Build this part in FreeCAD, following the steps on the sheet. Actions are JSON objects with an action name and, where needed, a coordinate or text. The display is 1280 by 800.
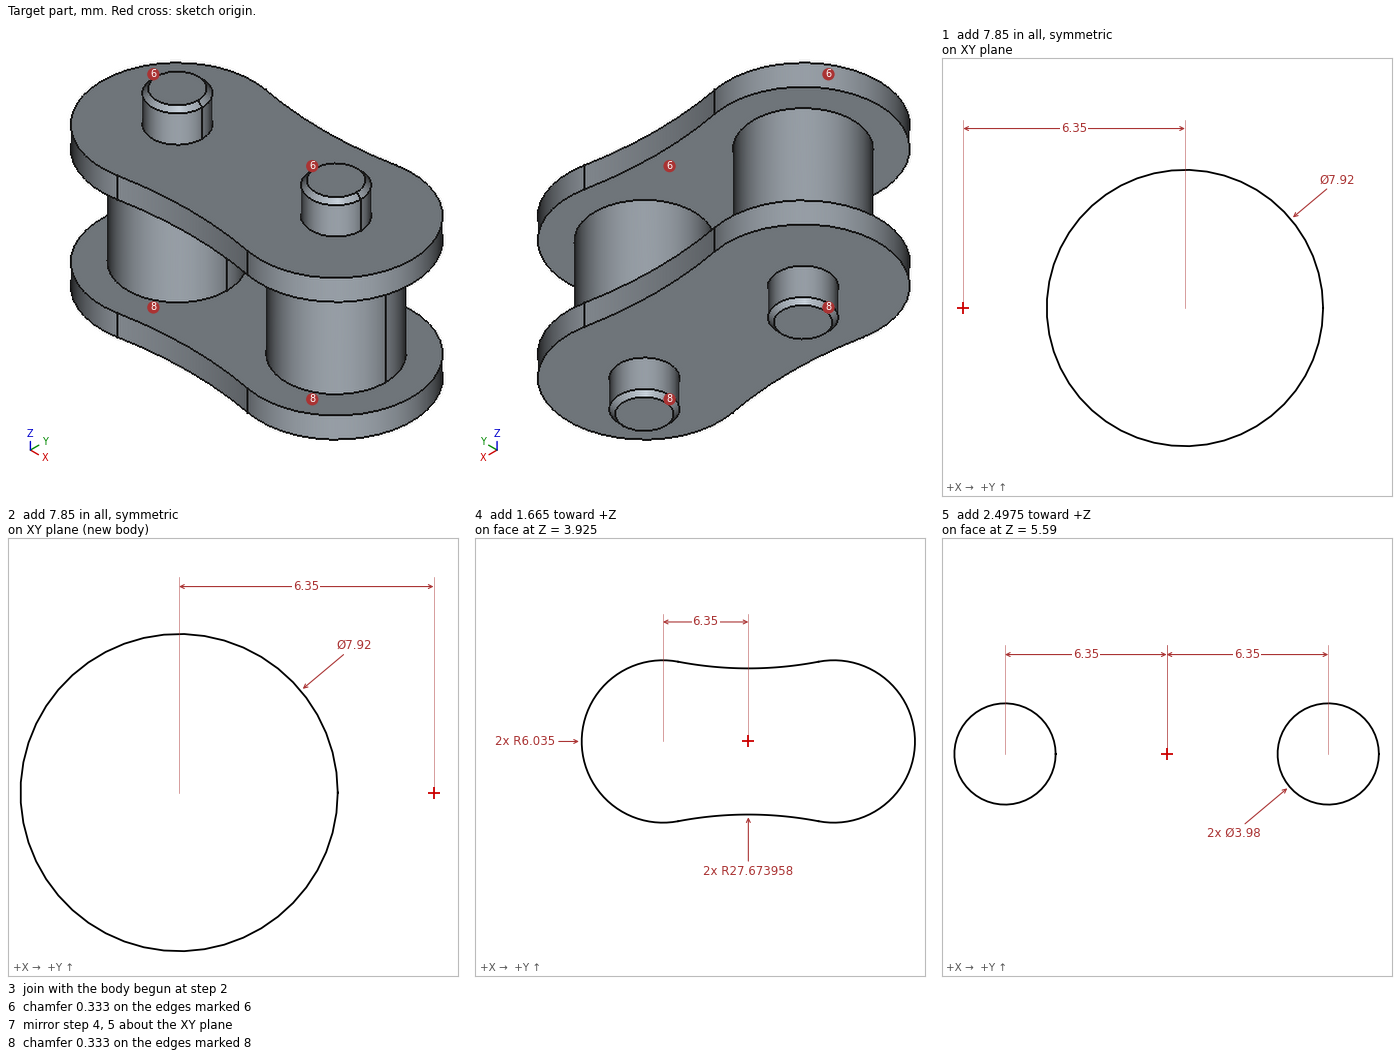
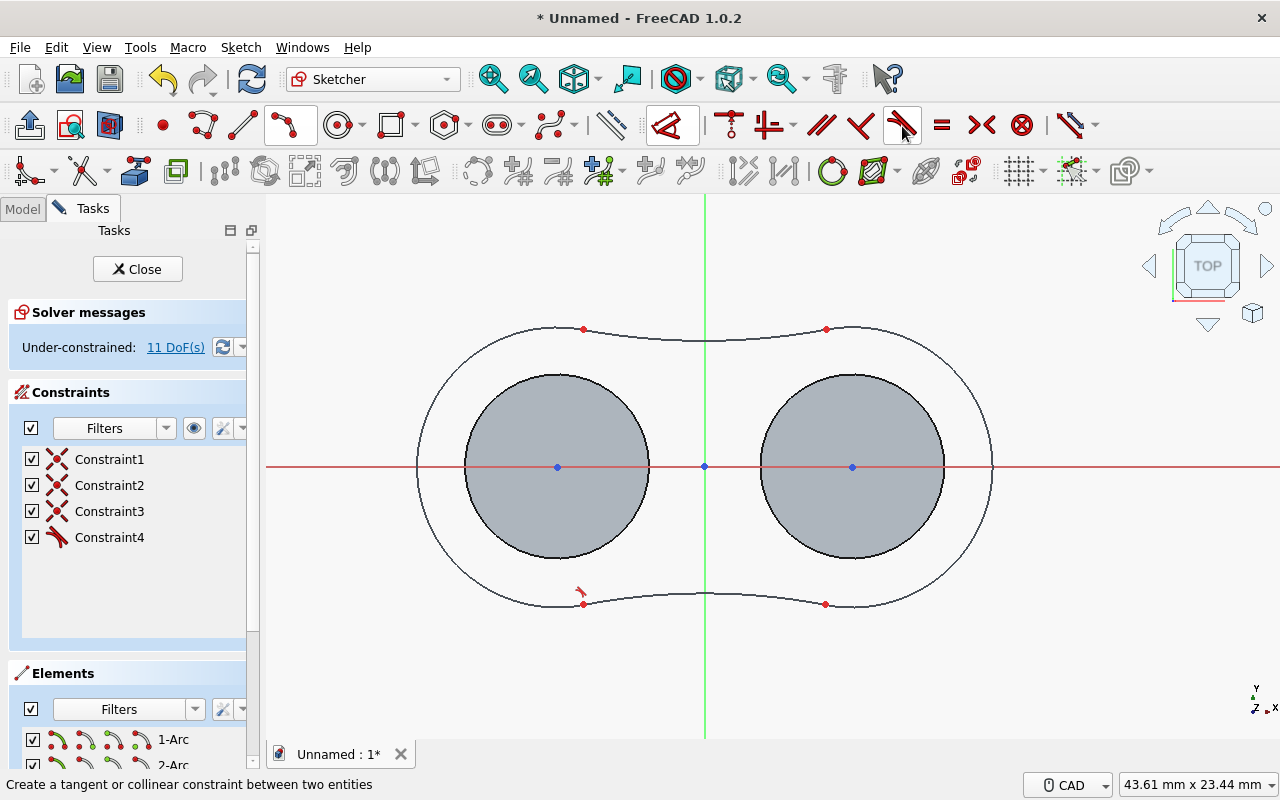
{"action": "left_click", "coordinate": [450, 377]}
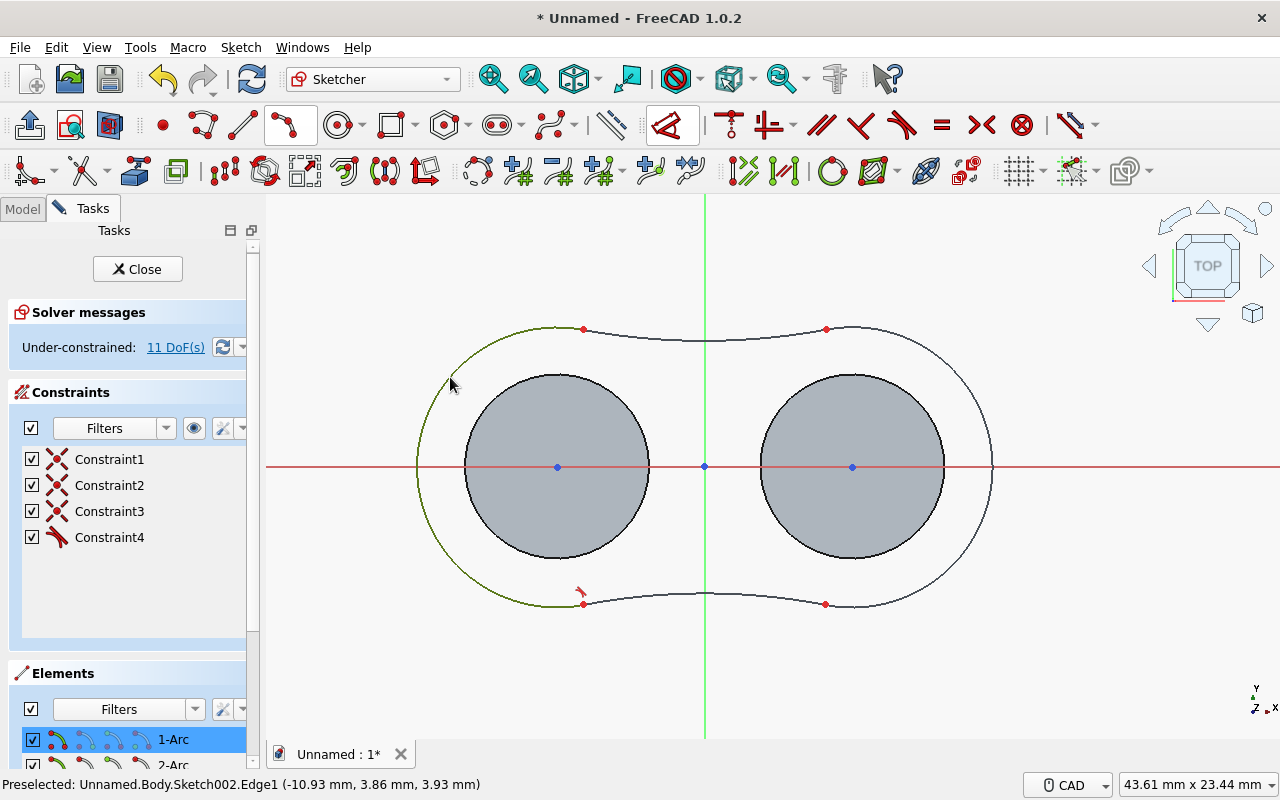
{"action": "left_click", "coordinate": [656, 339]}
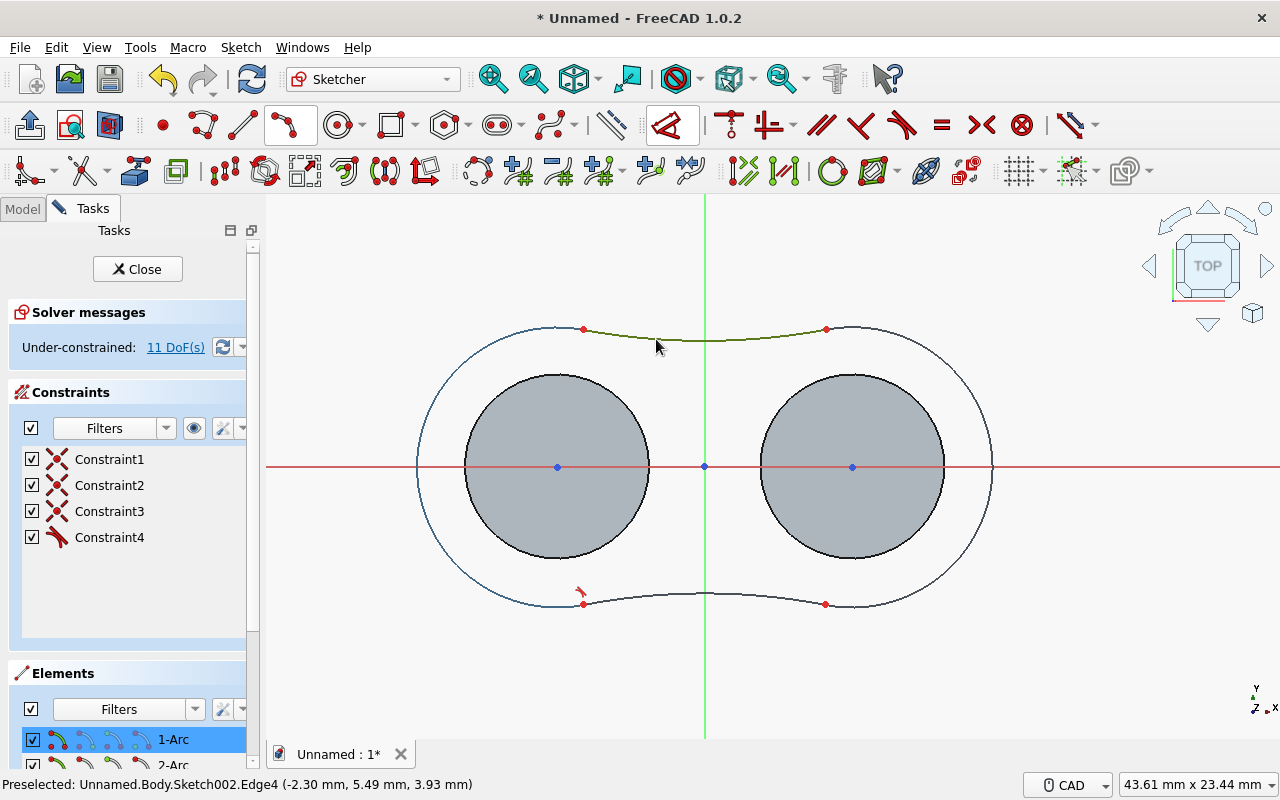
{"action": "key", "text": "t"}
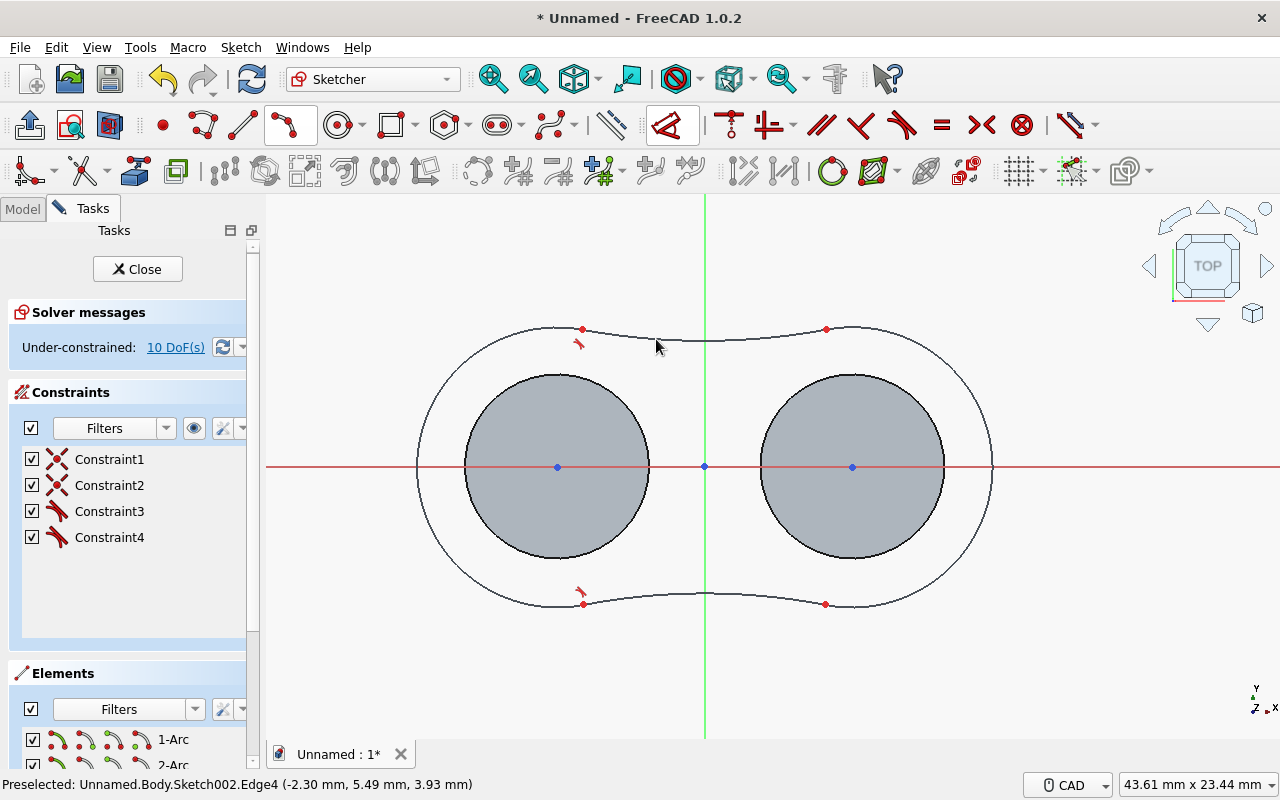
{"action": "left_click", "coordinate": [753, 595]}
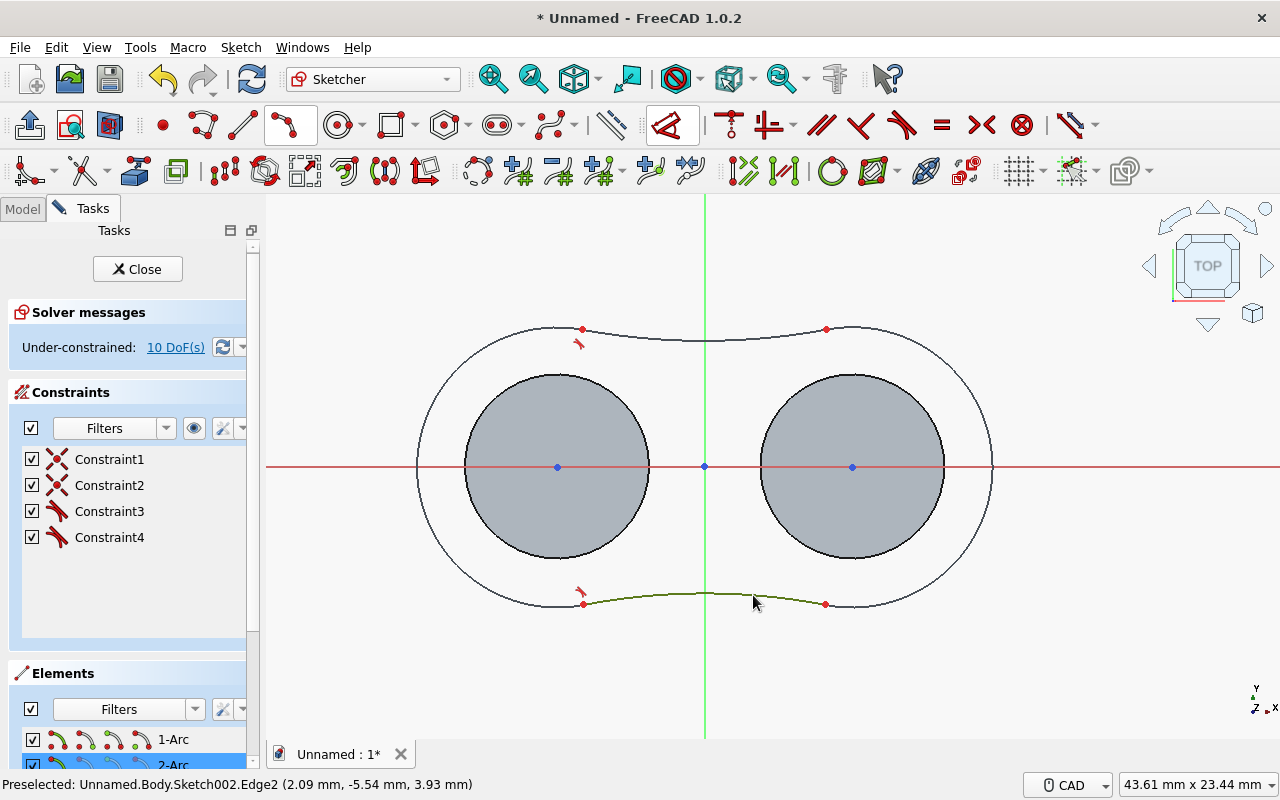
{"action": "left_click", "coordinate": [959, 558]}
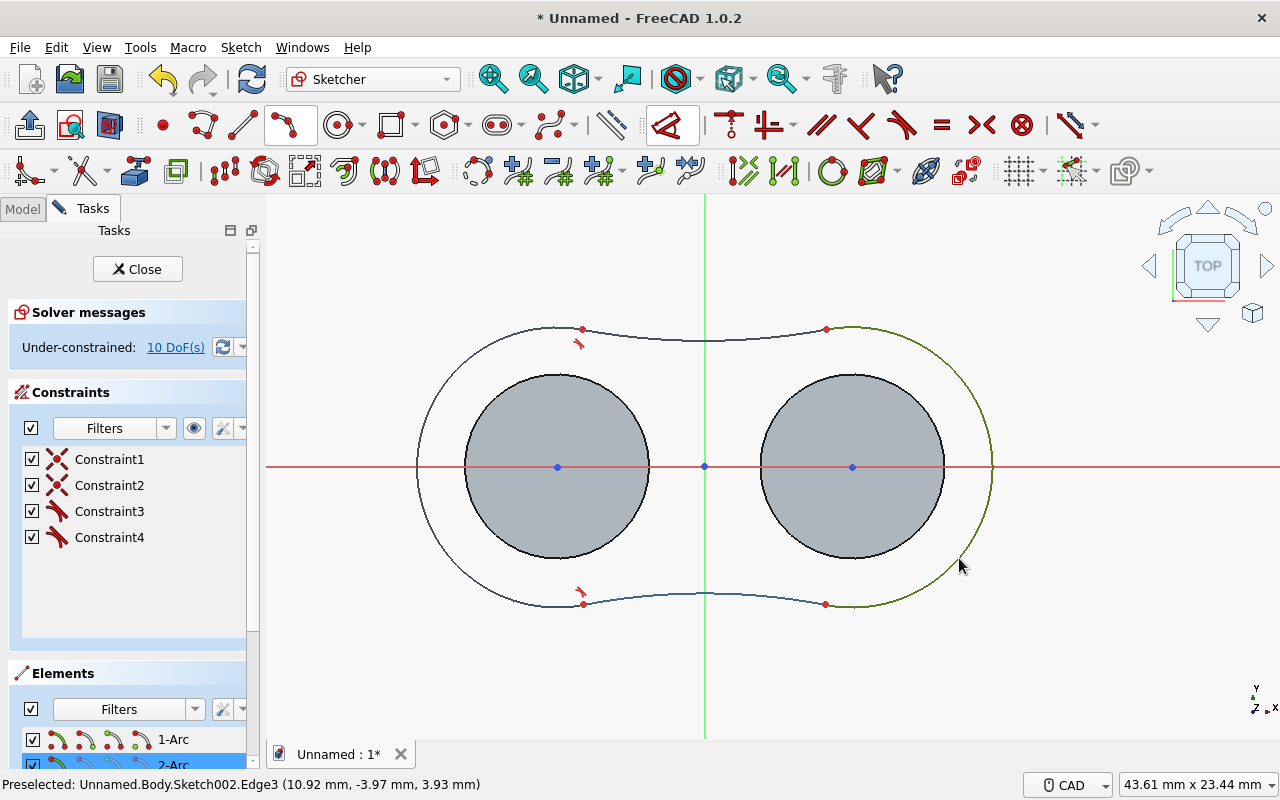
{"action": "key", "text": "t"}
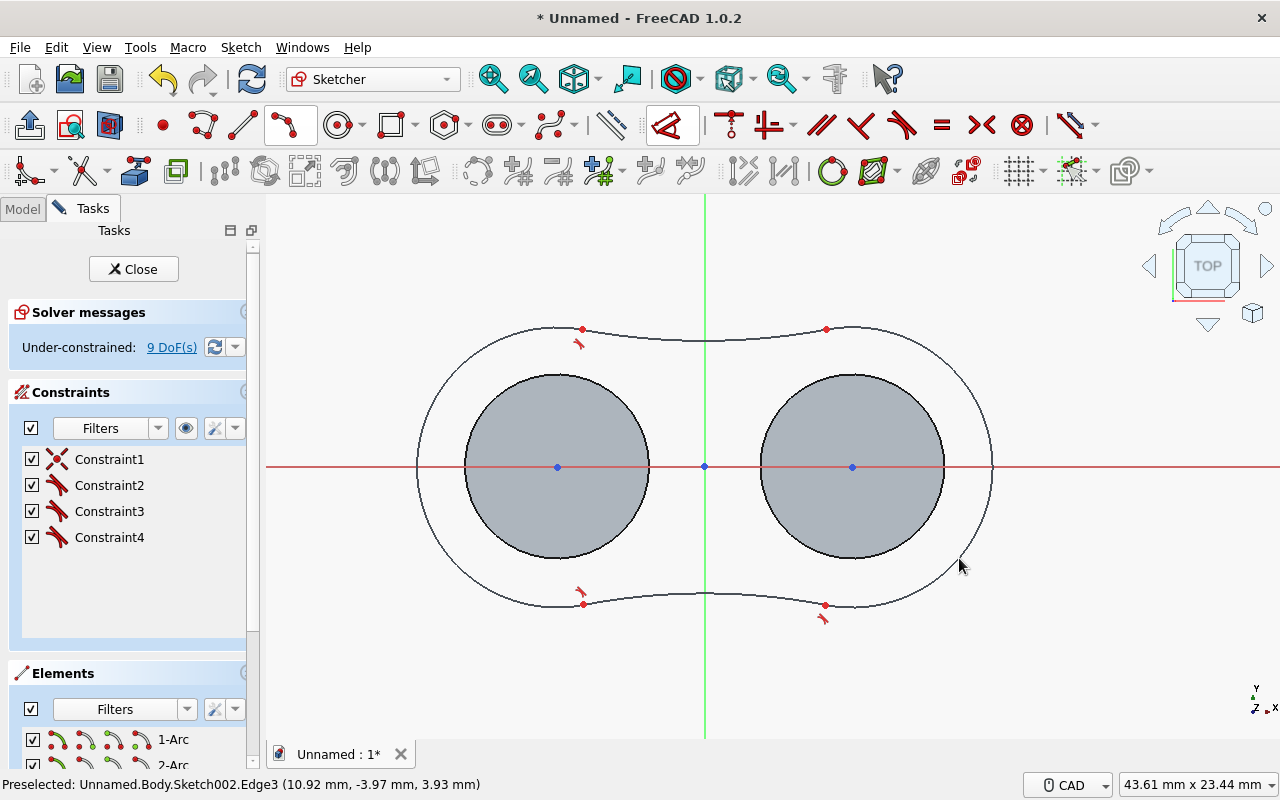
{"action": "left_click", "coordinate": [959, 558]}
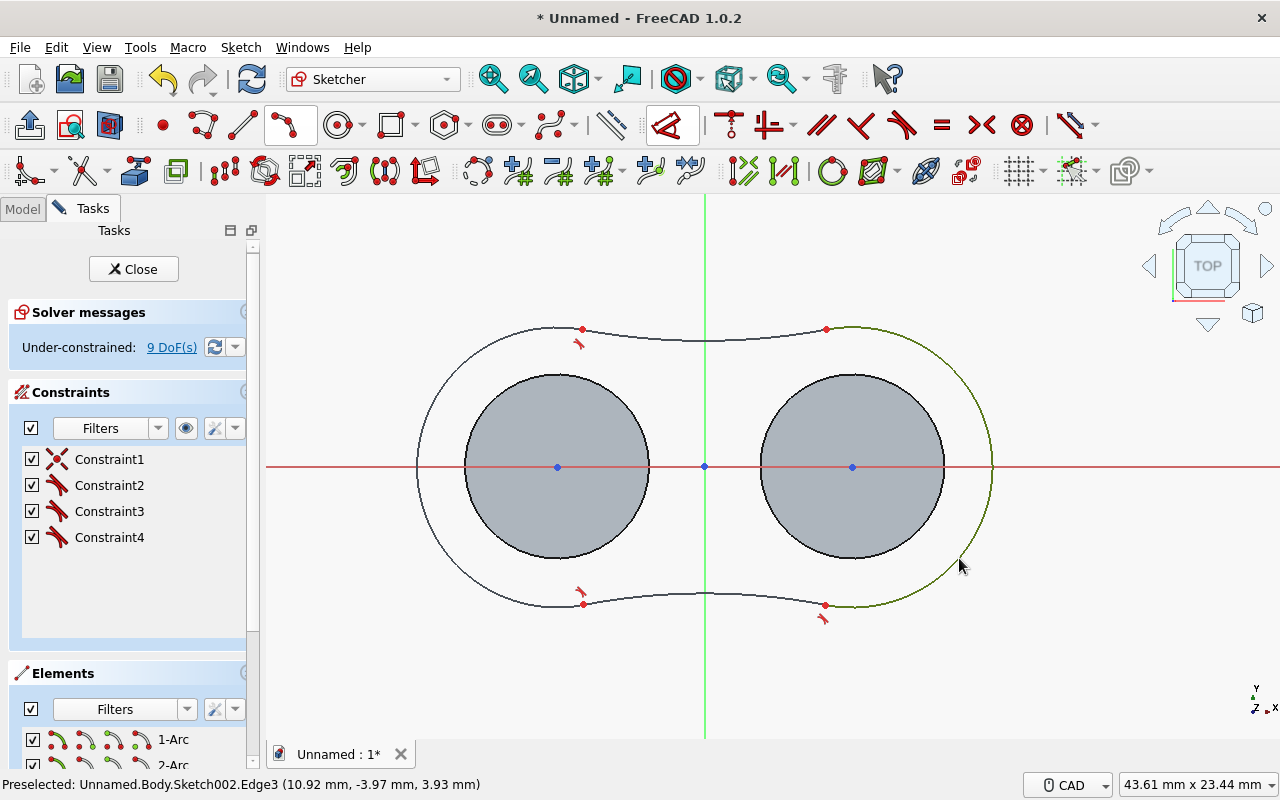
{"action": "left_click", "coordinate": [655, 339]}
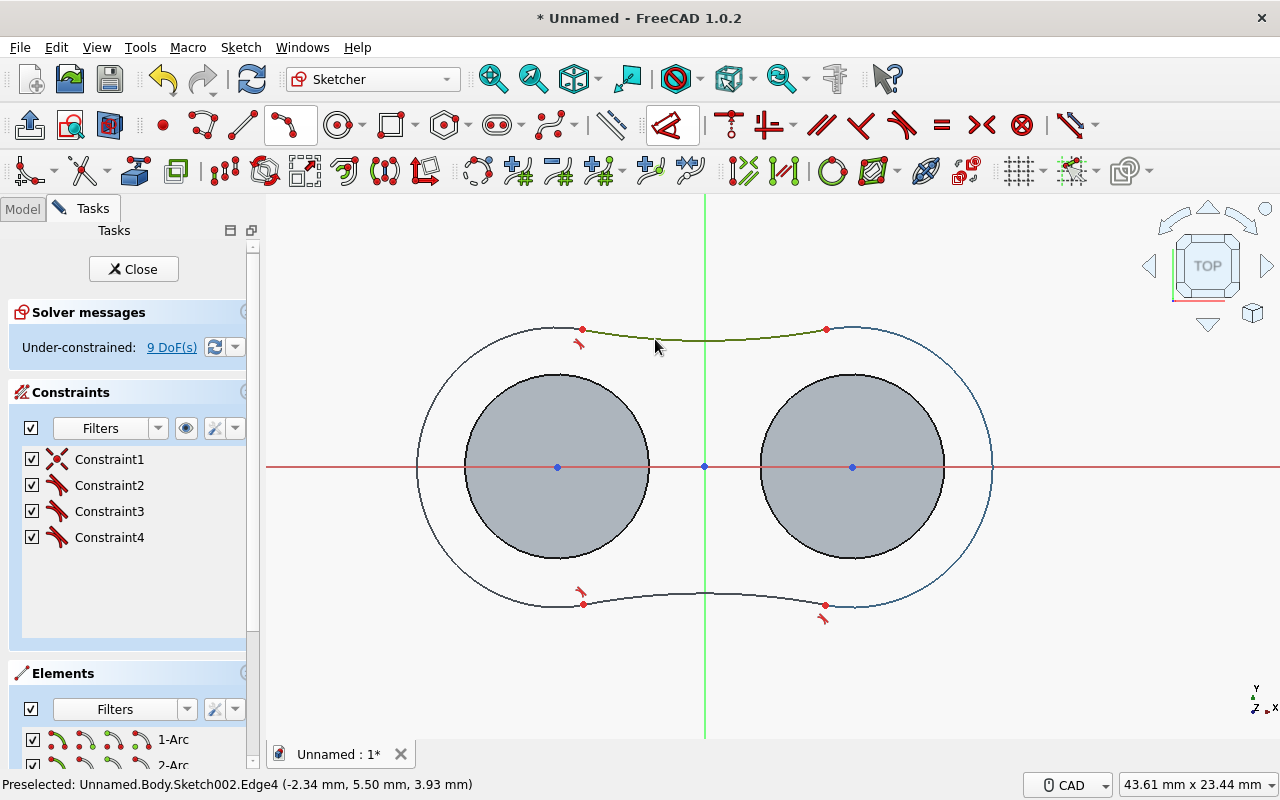
{"action": "left_click", "coordinate": [902, 126]}